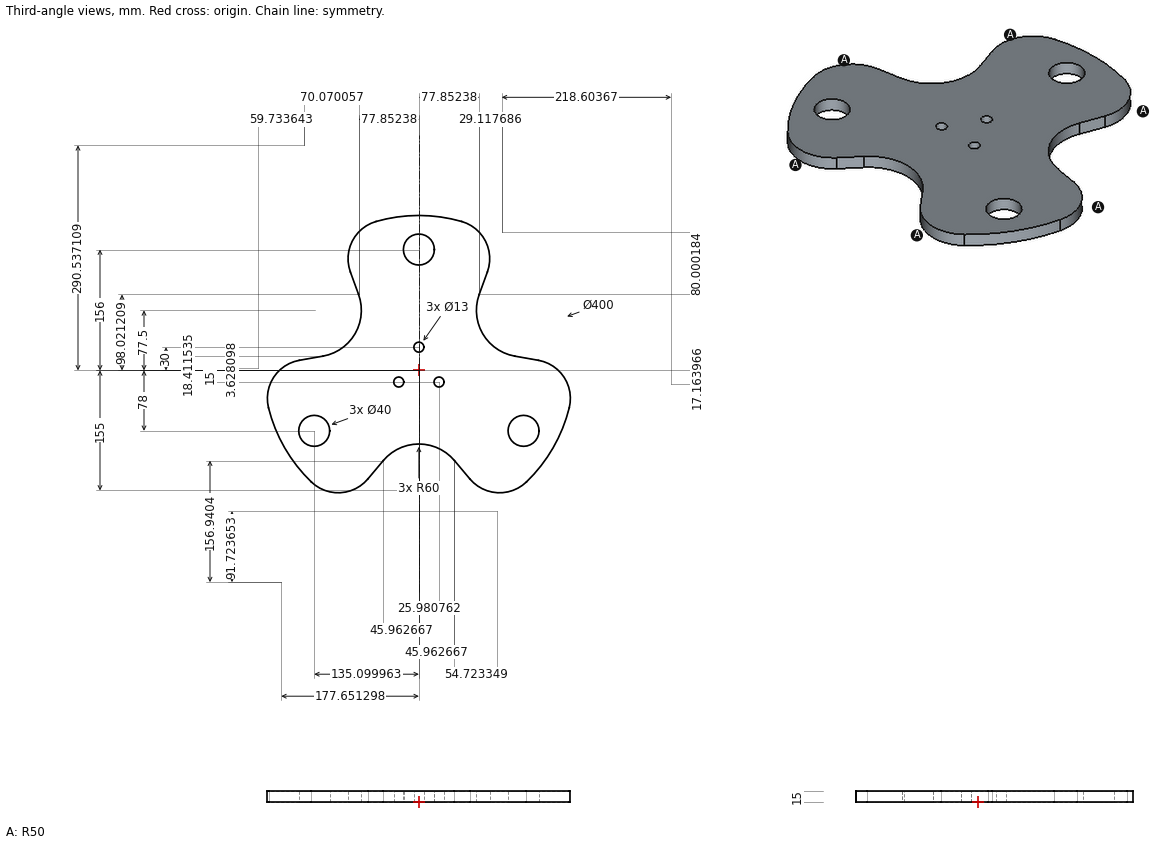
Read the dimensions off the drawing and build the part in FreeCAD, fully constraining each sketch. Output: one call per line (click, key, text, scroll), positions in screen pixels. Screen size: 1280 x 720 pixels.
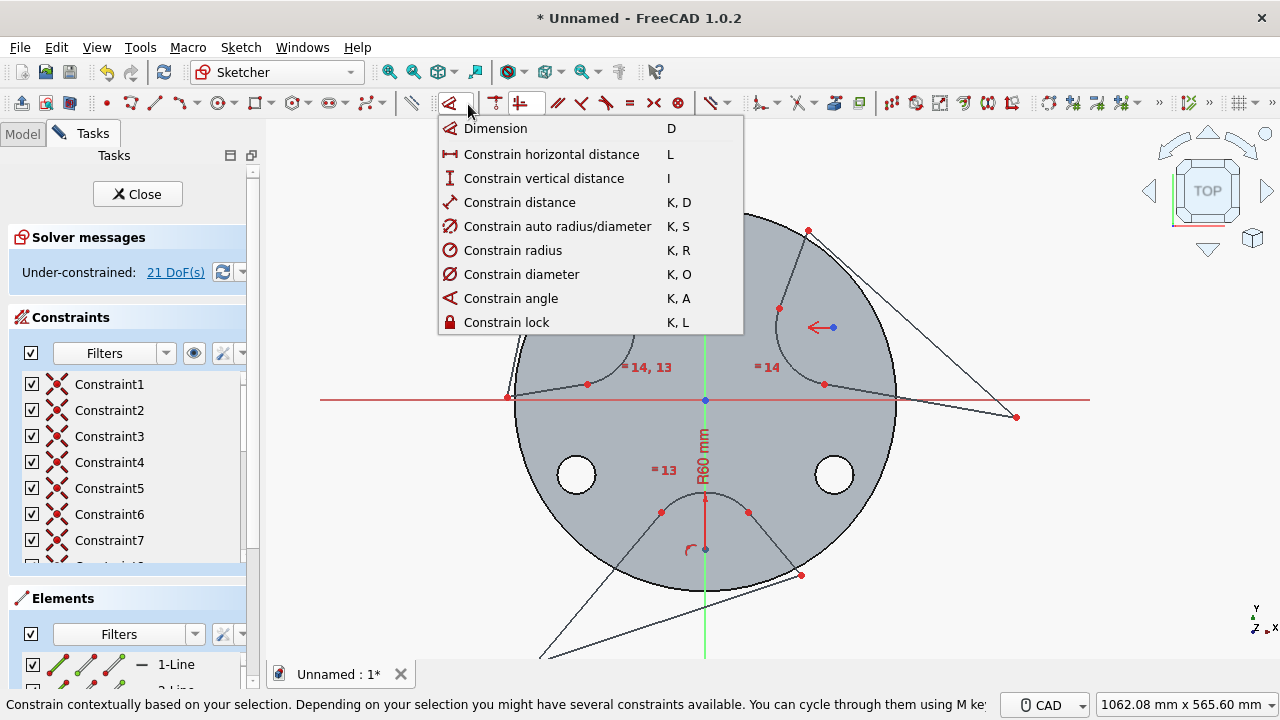
click(591, 178)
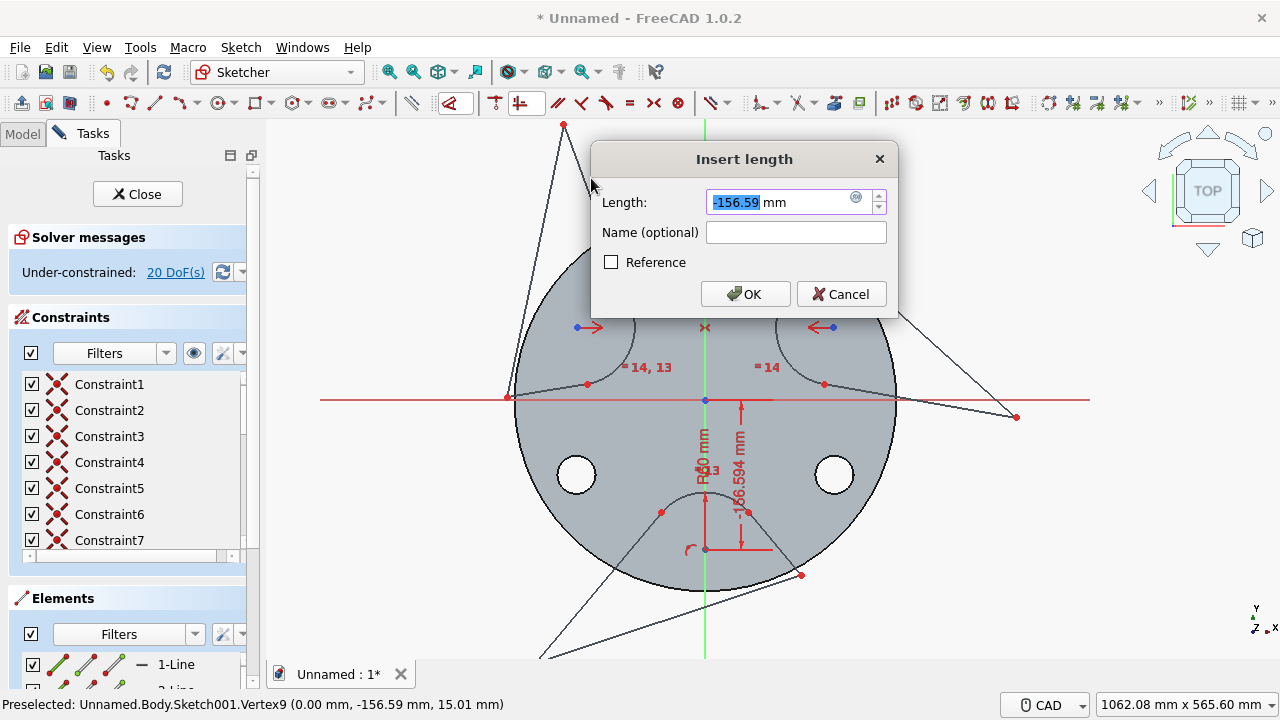
text(-155)
key(Return)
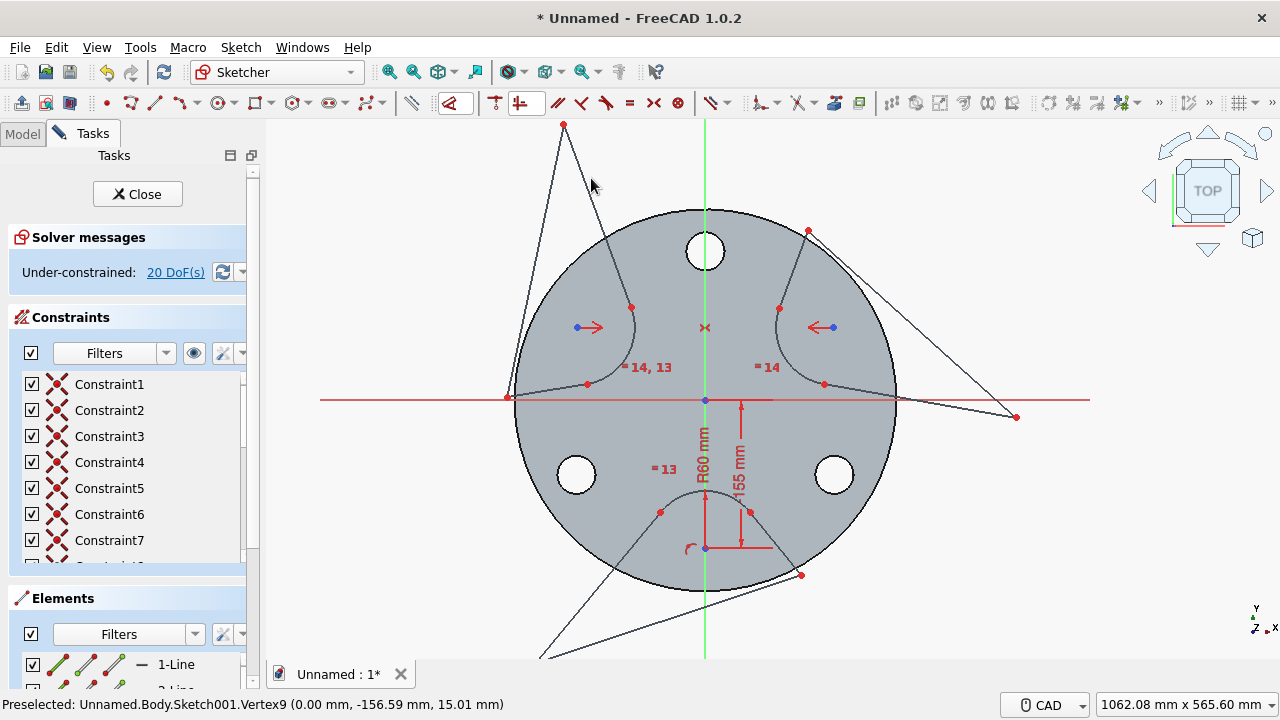
click(577, 328)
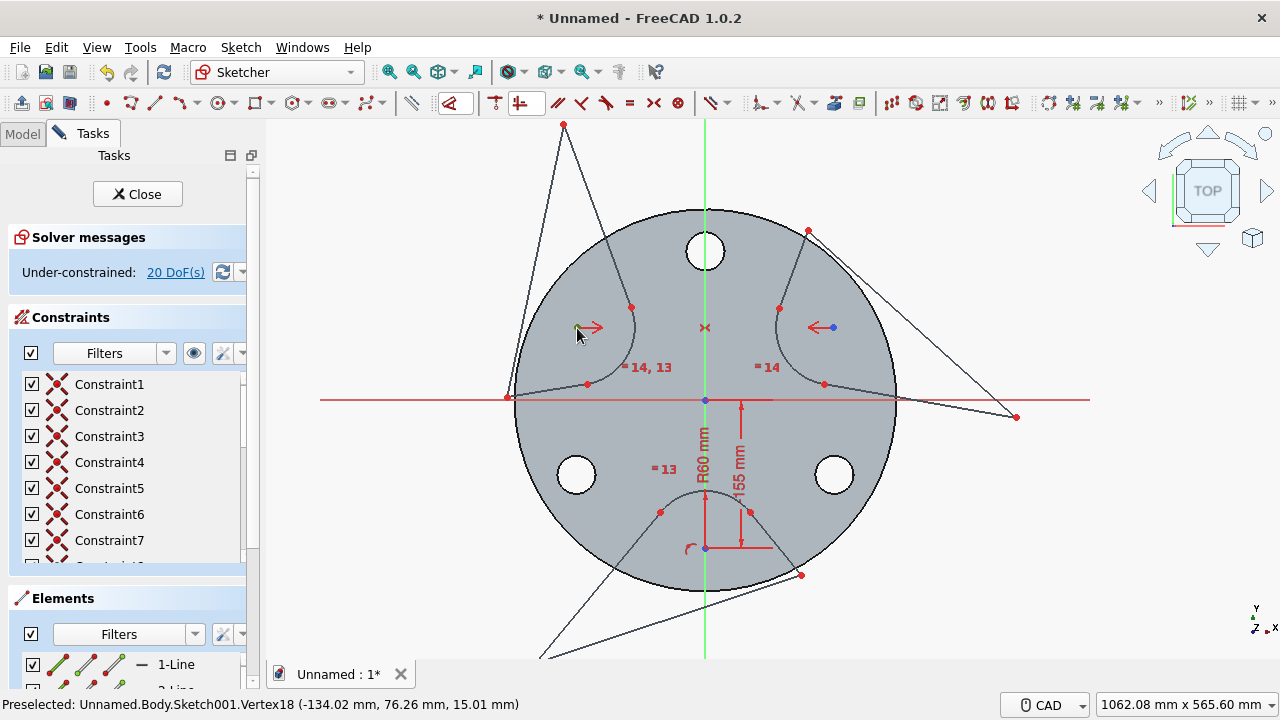
click(468, 104)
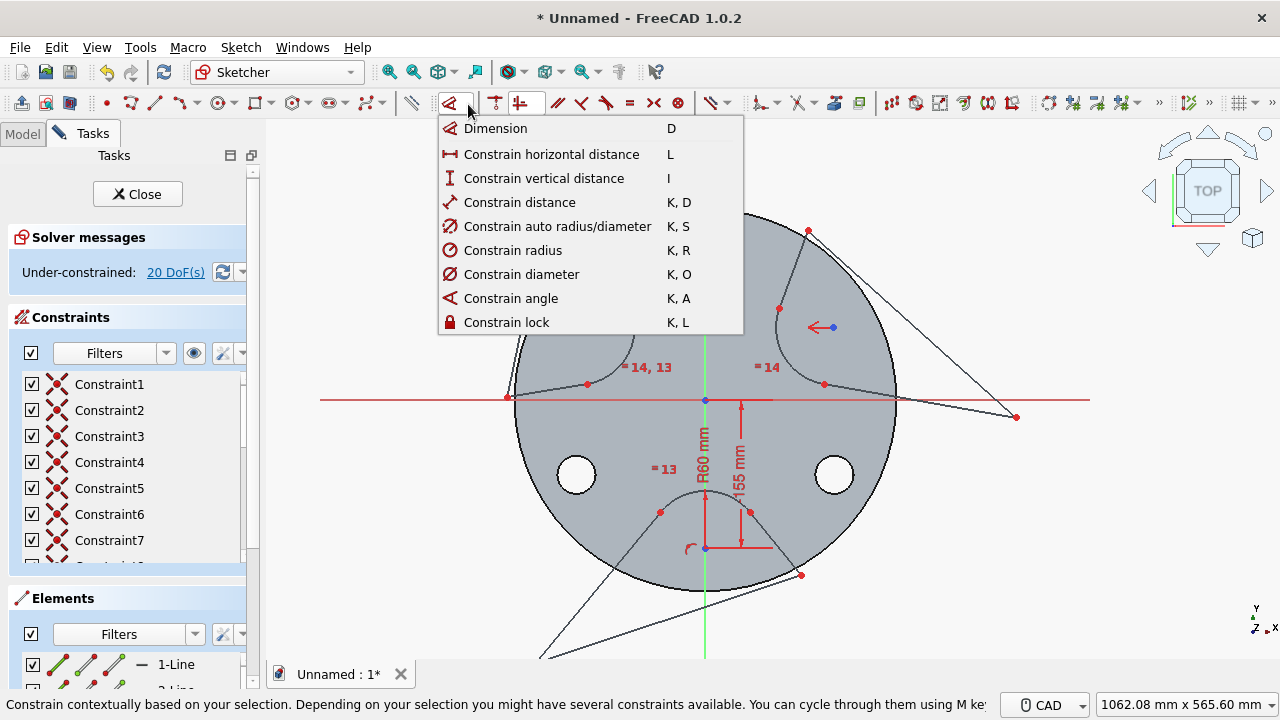
click(591, 178)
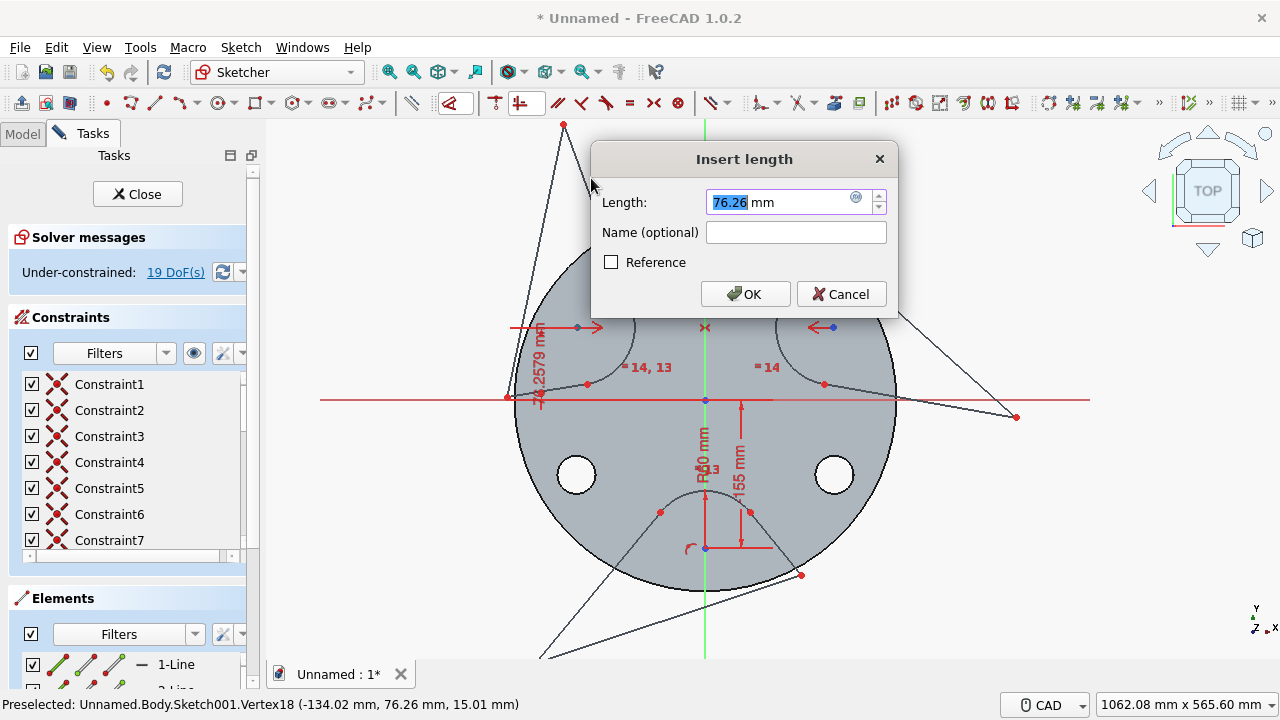
text(77.5)
key(Return)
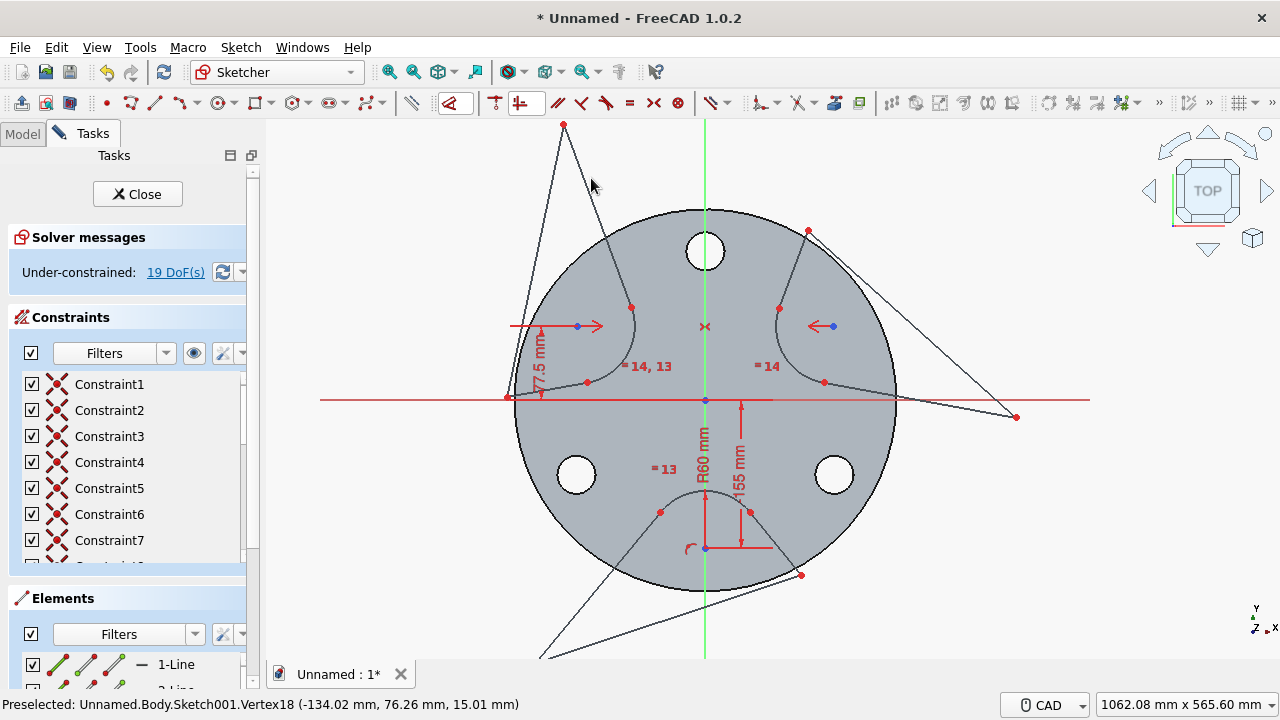
click(632, 308)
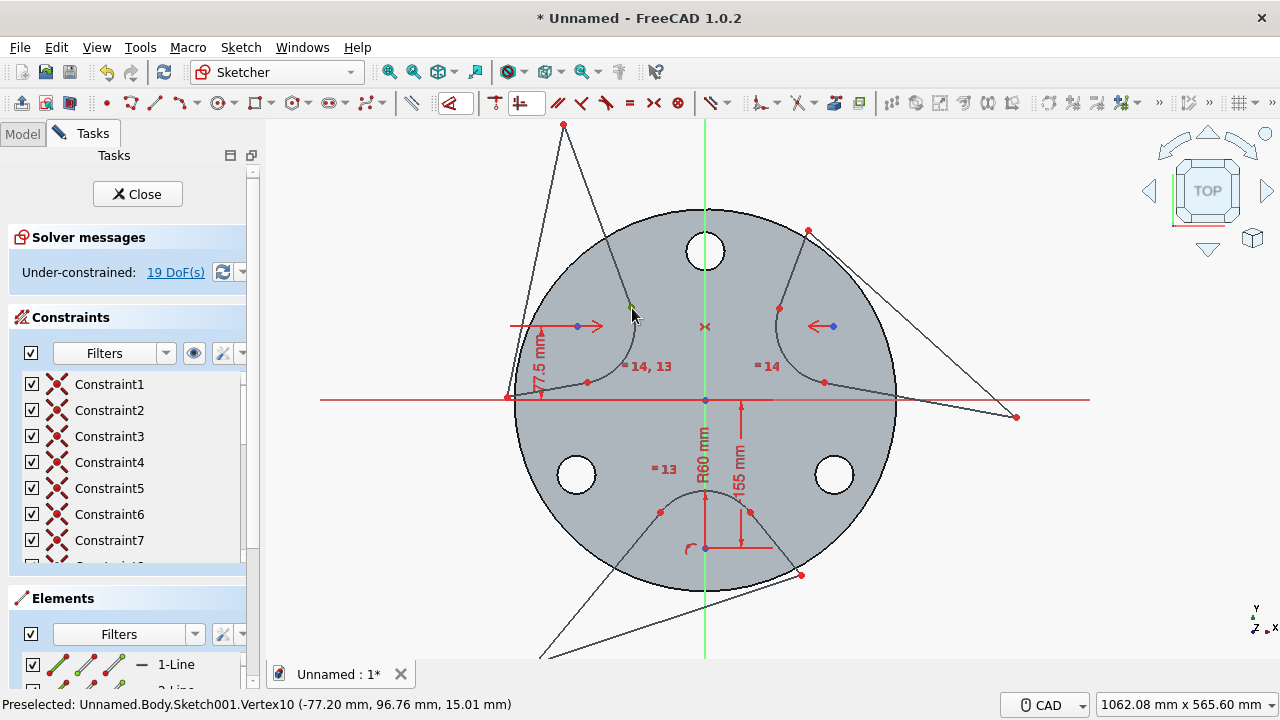
click(468, 104)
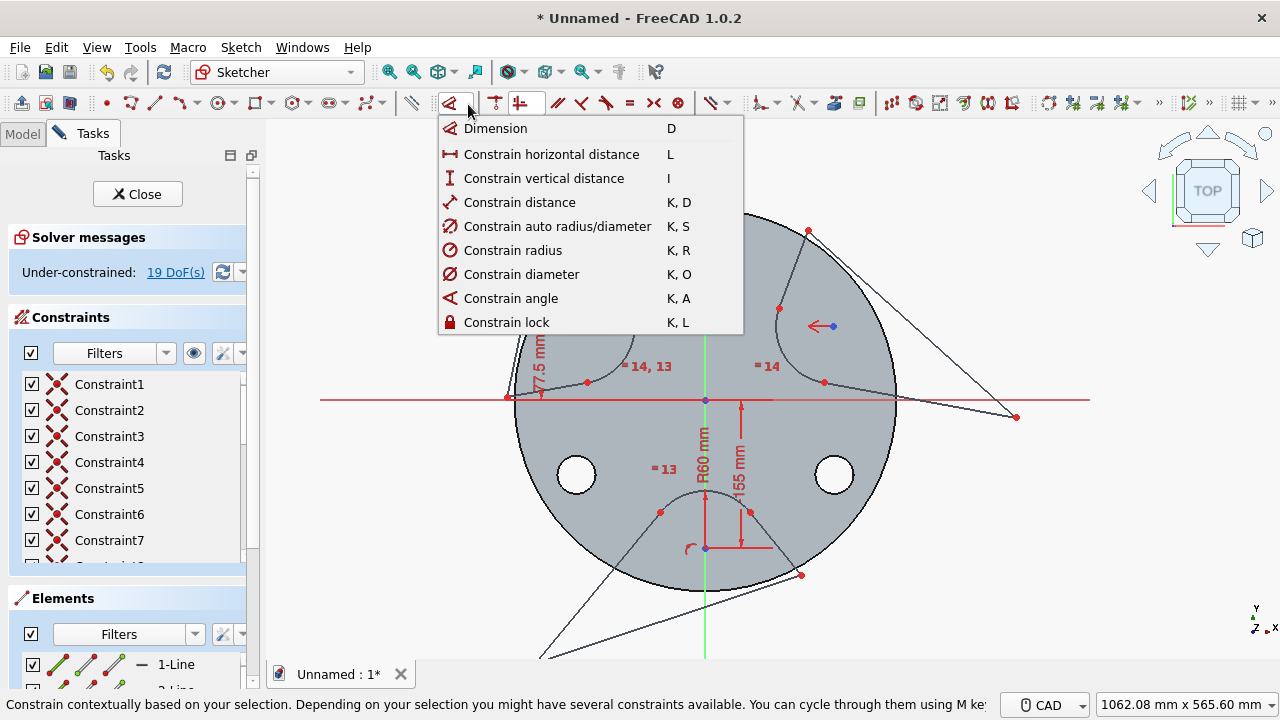
click(591, 154)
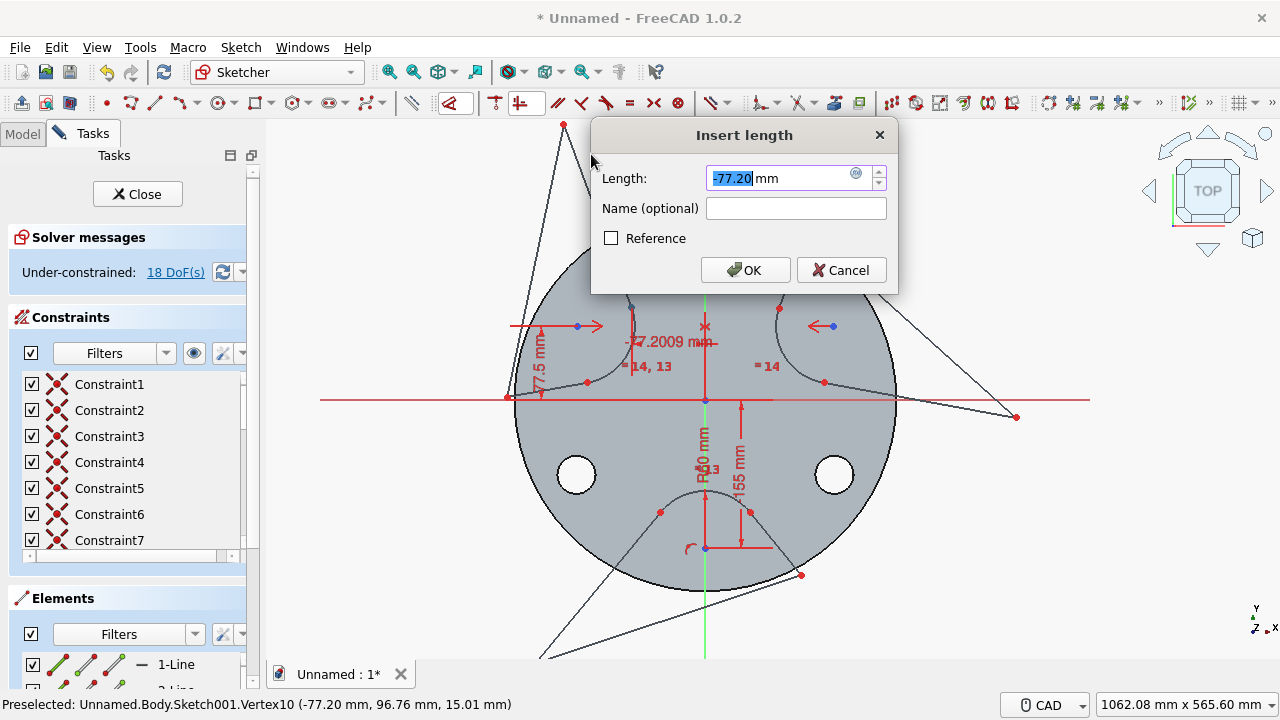
text(-77.85238)
key(Return)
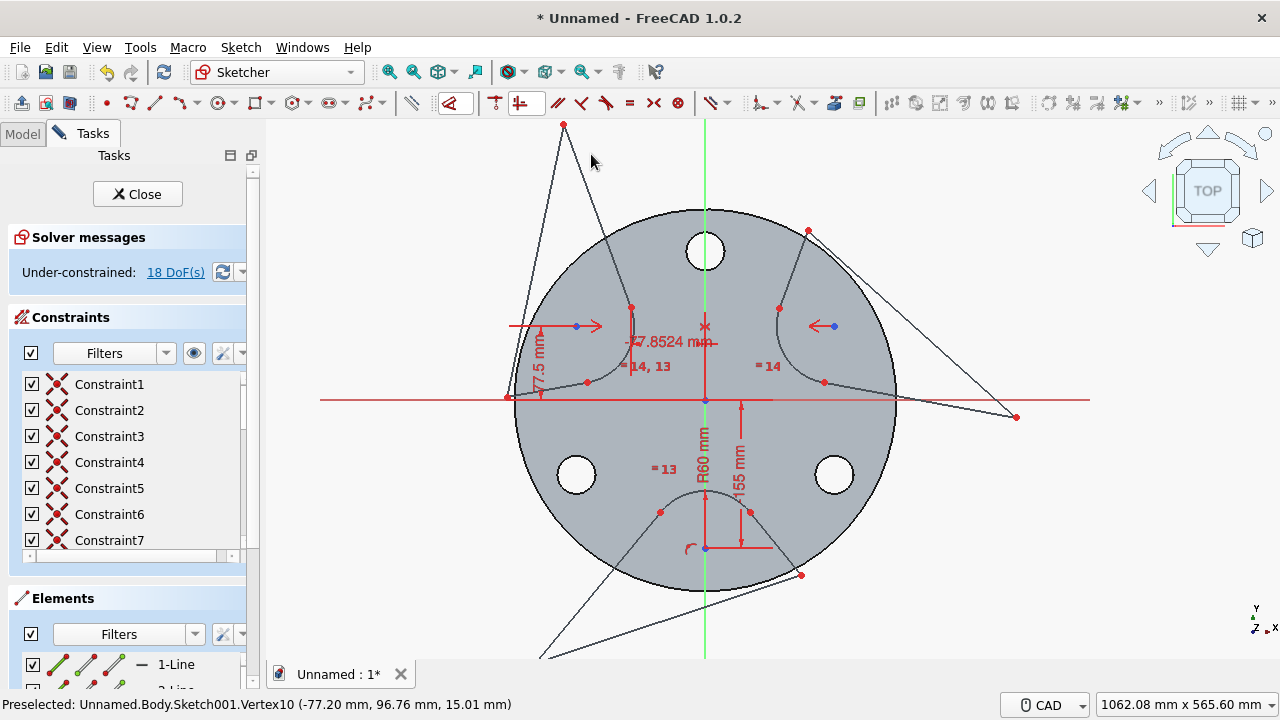
scroll(507, 397, up, 13)